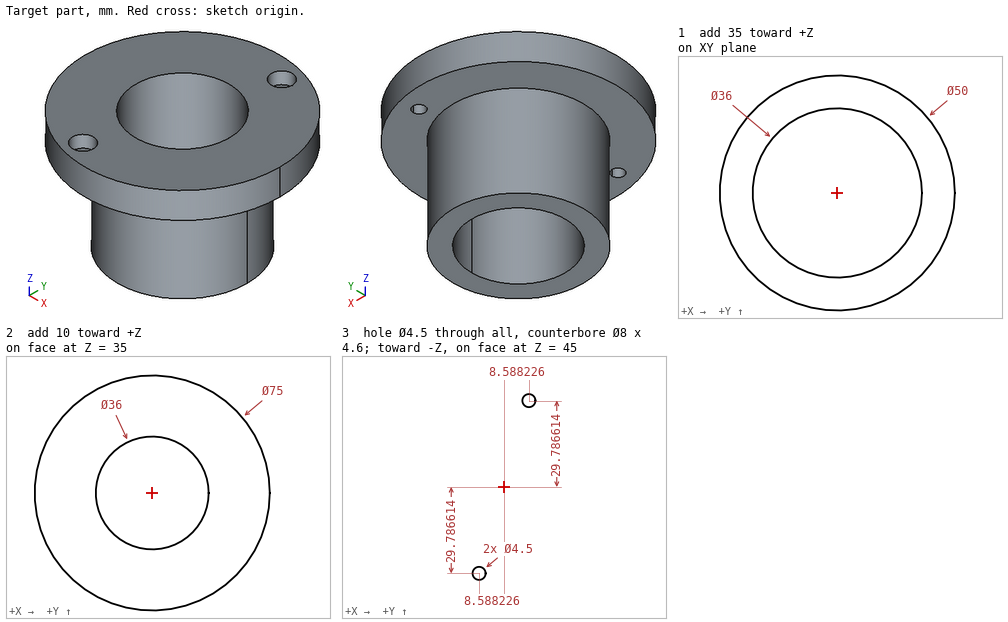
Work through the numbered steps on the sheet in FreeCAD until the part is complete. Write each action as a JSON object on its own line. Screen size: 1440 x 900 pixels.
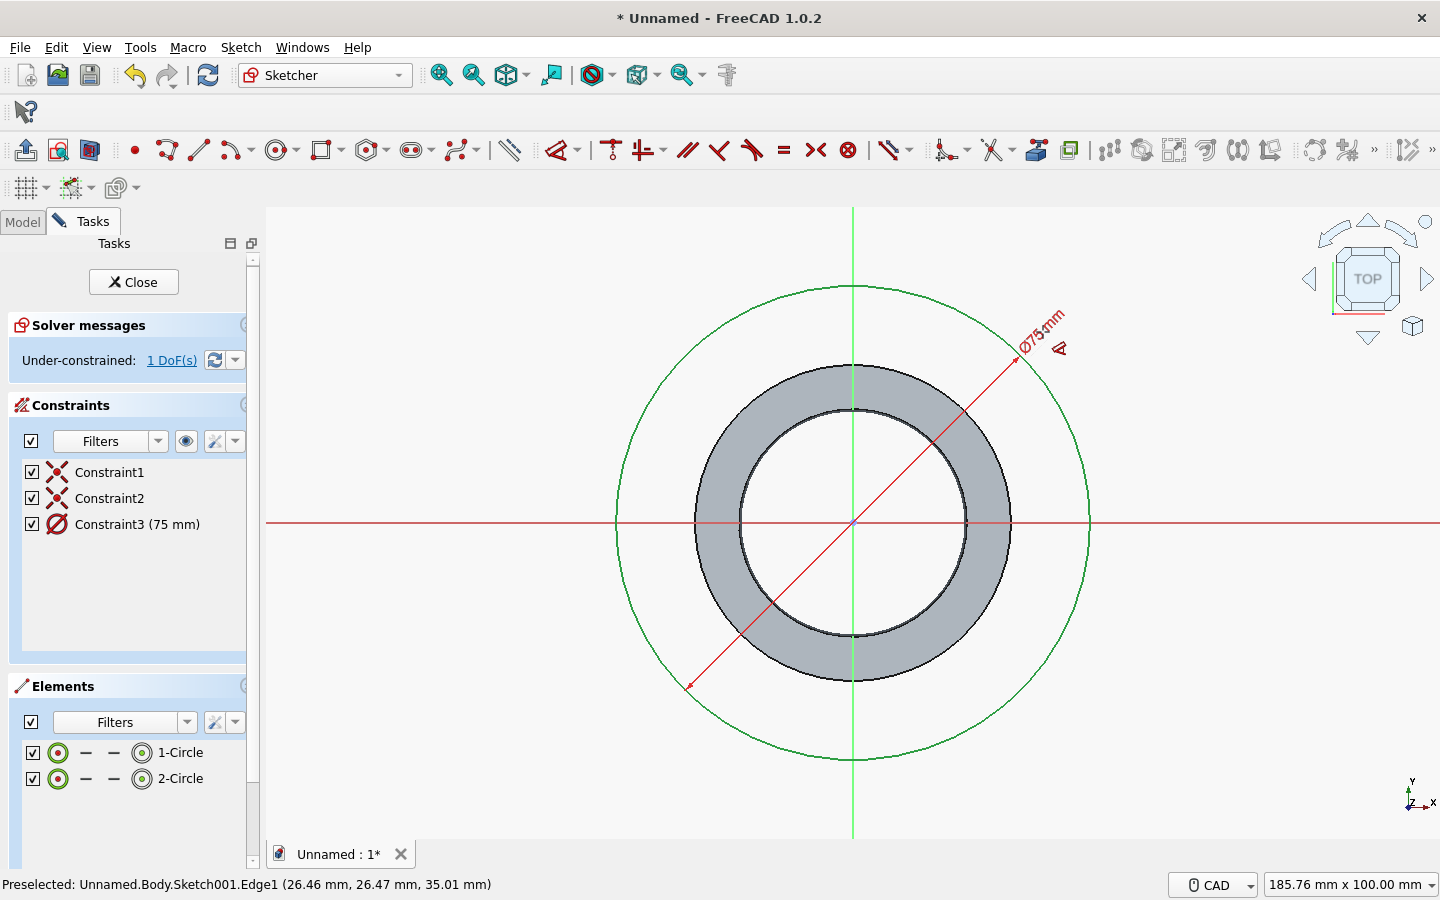
{"action": "left_click", "coordinate": [932, 443]}
{"action": "left_click", "coordinate": [954, 420]}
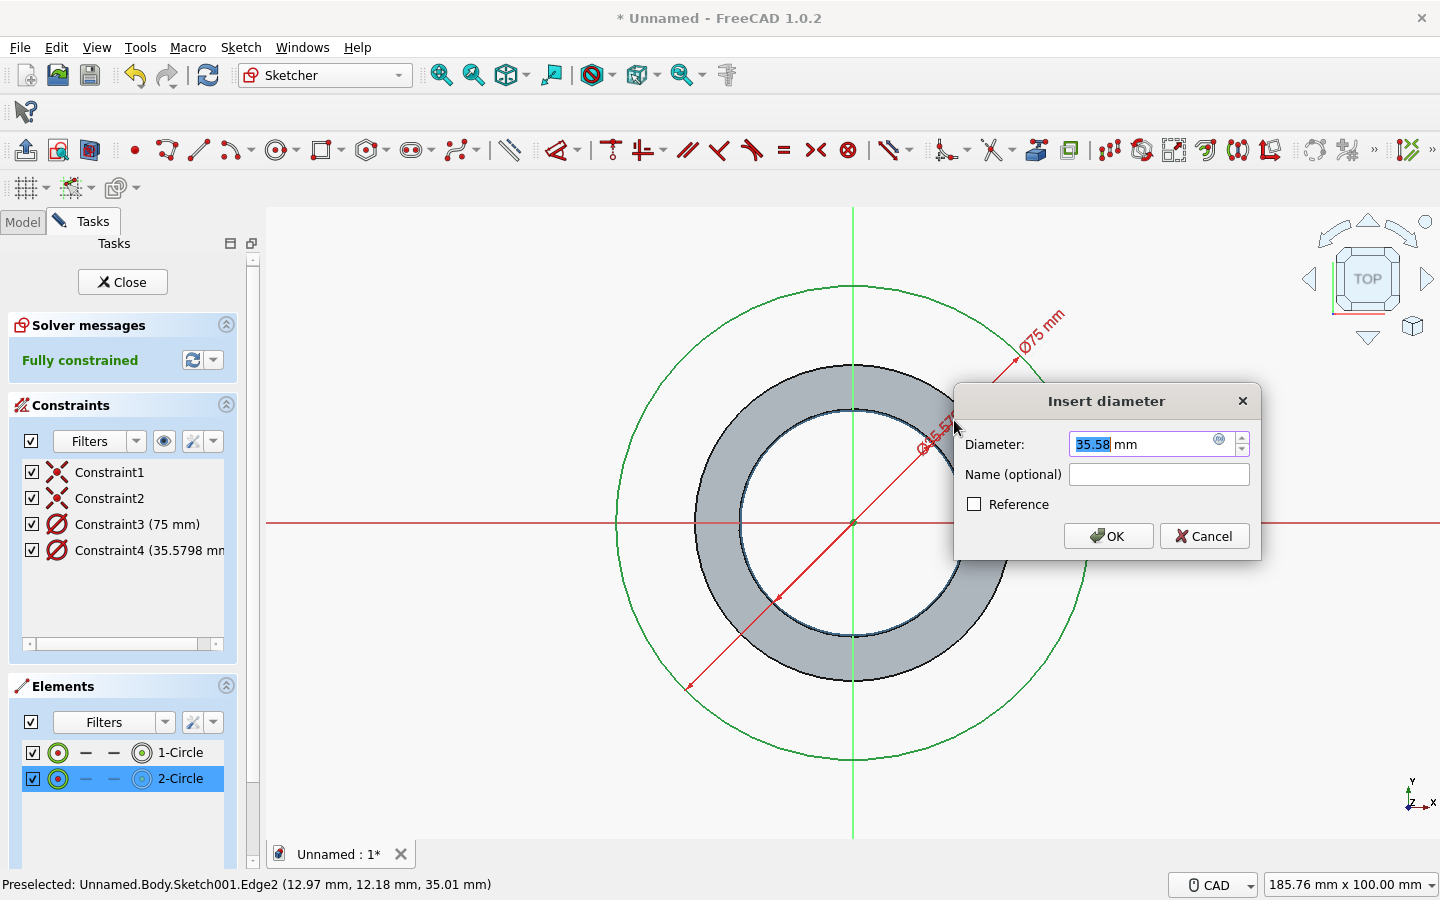
{"action": "type", "text": "36"}
{"action": "key", "text": "Return"}
{"action": "key", "text": "Escape"}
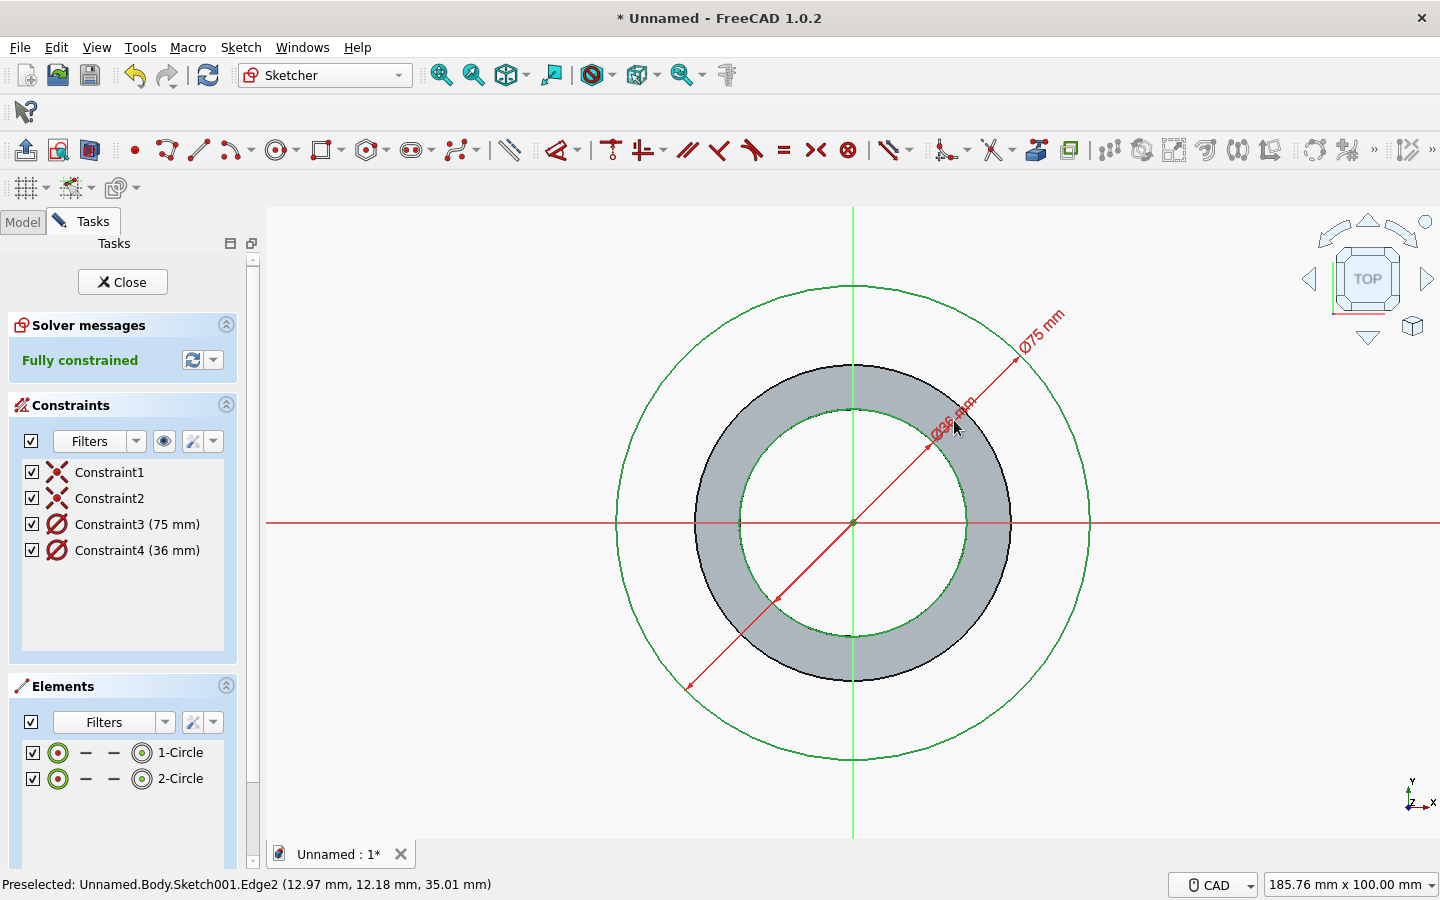
{"action": "left_click", "coordinate": [123, 282]}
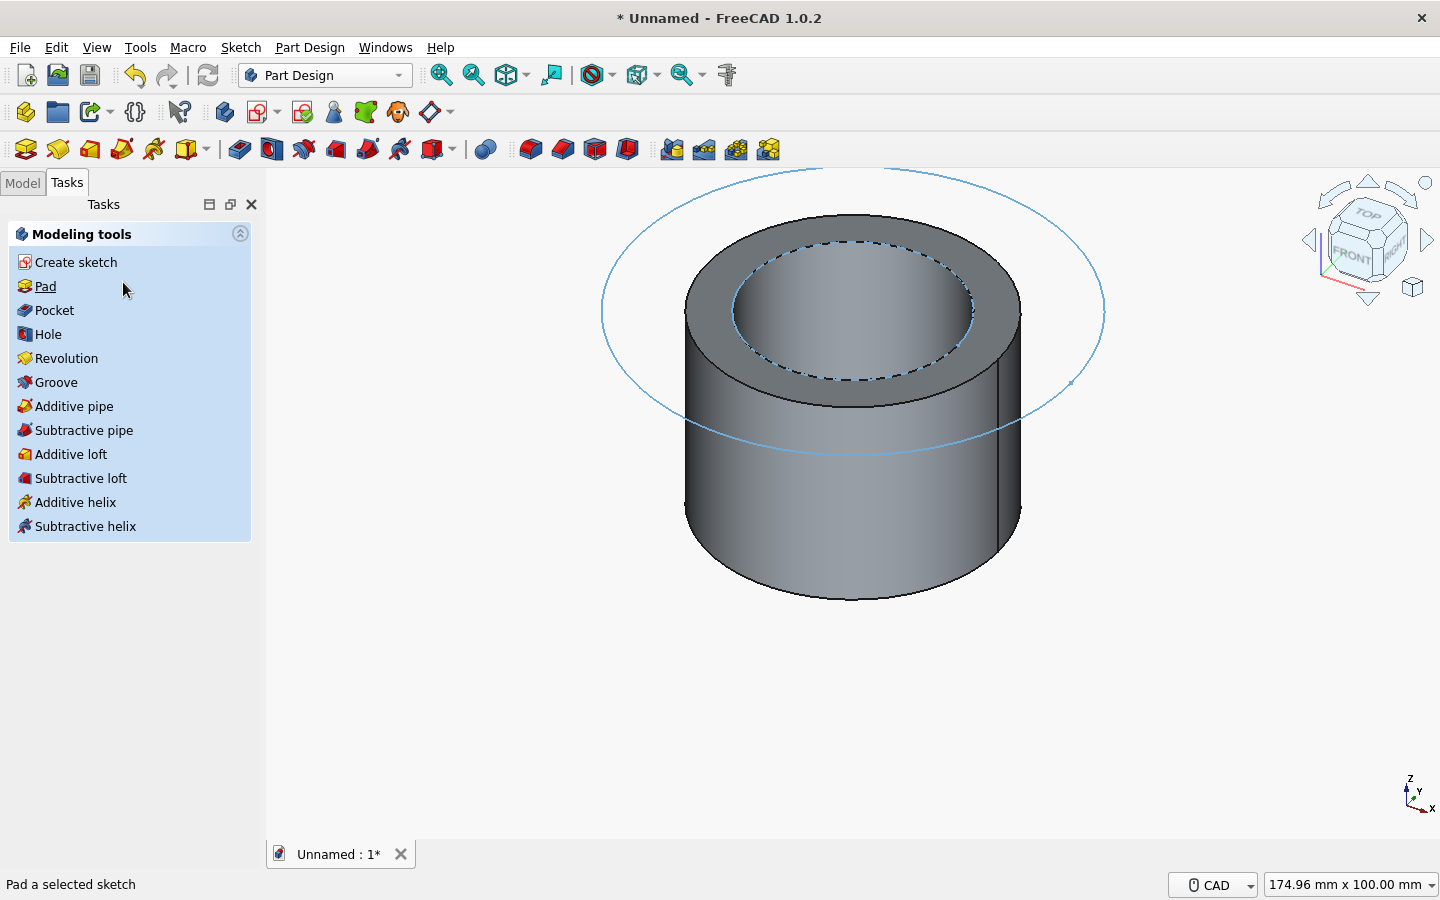
{"action": "left_click", "coordinate": [26, 150]}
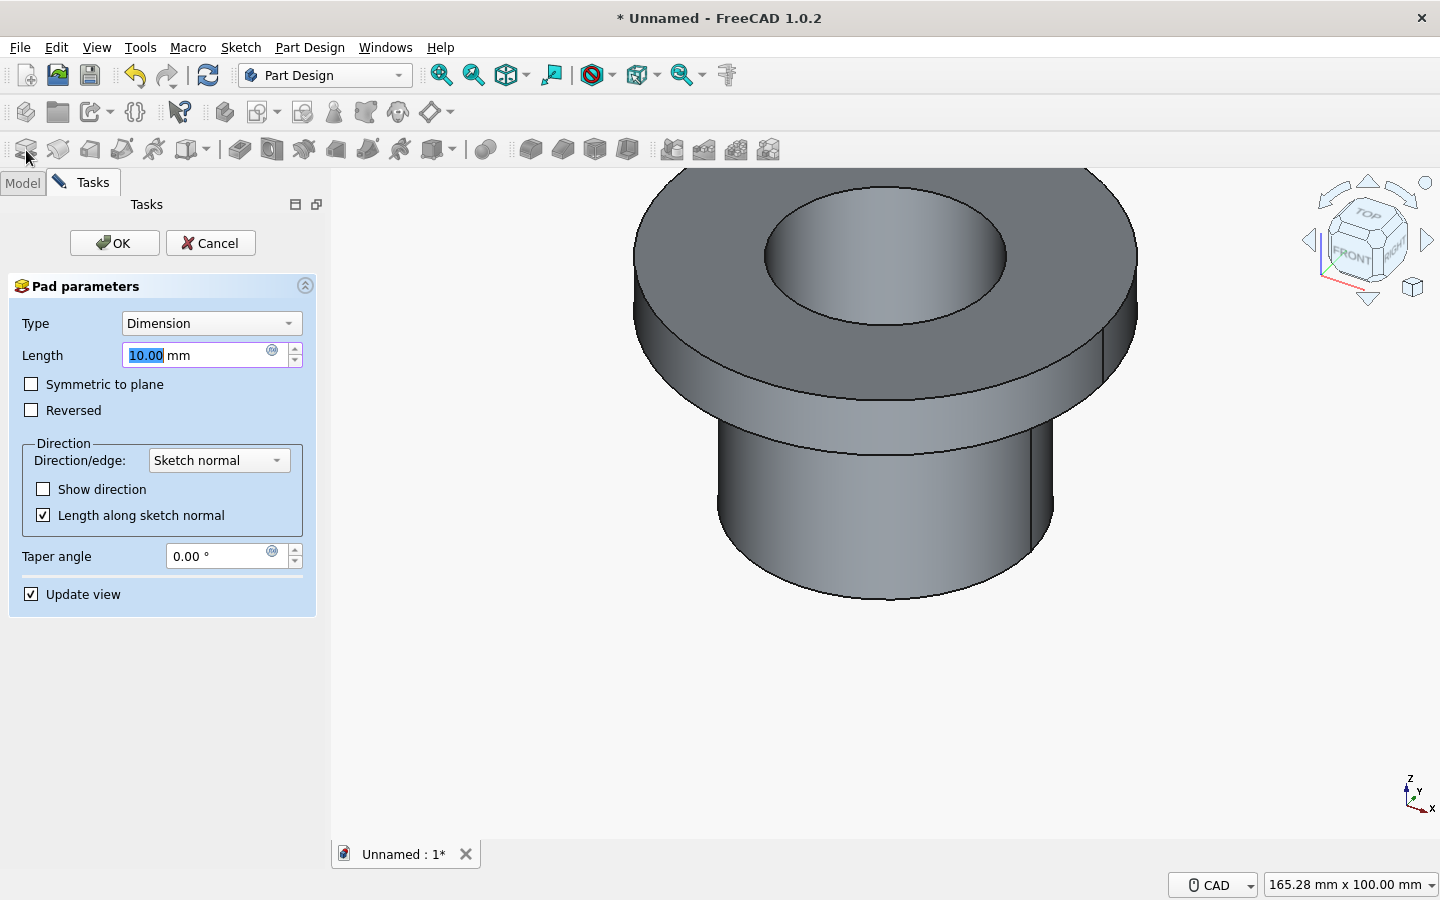
{"action": "type", "text": "10"}
{"action": "key", "text": "Tab"}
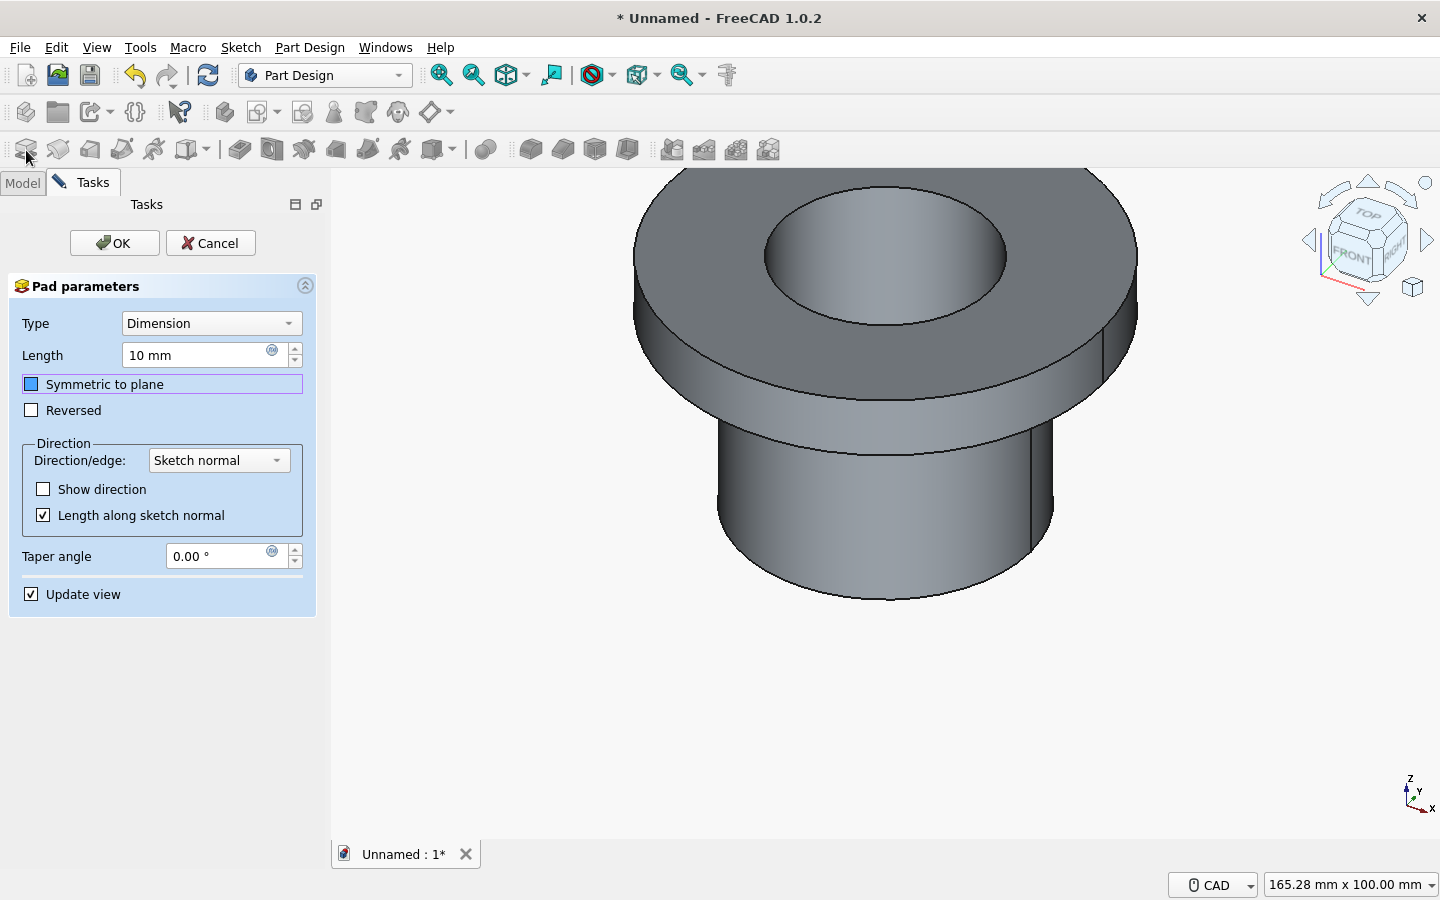
{"action": "left_click", "coordinate": [115, 243]}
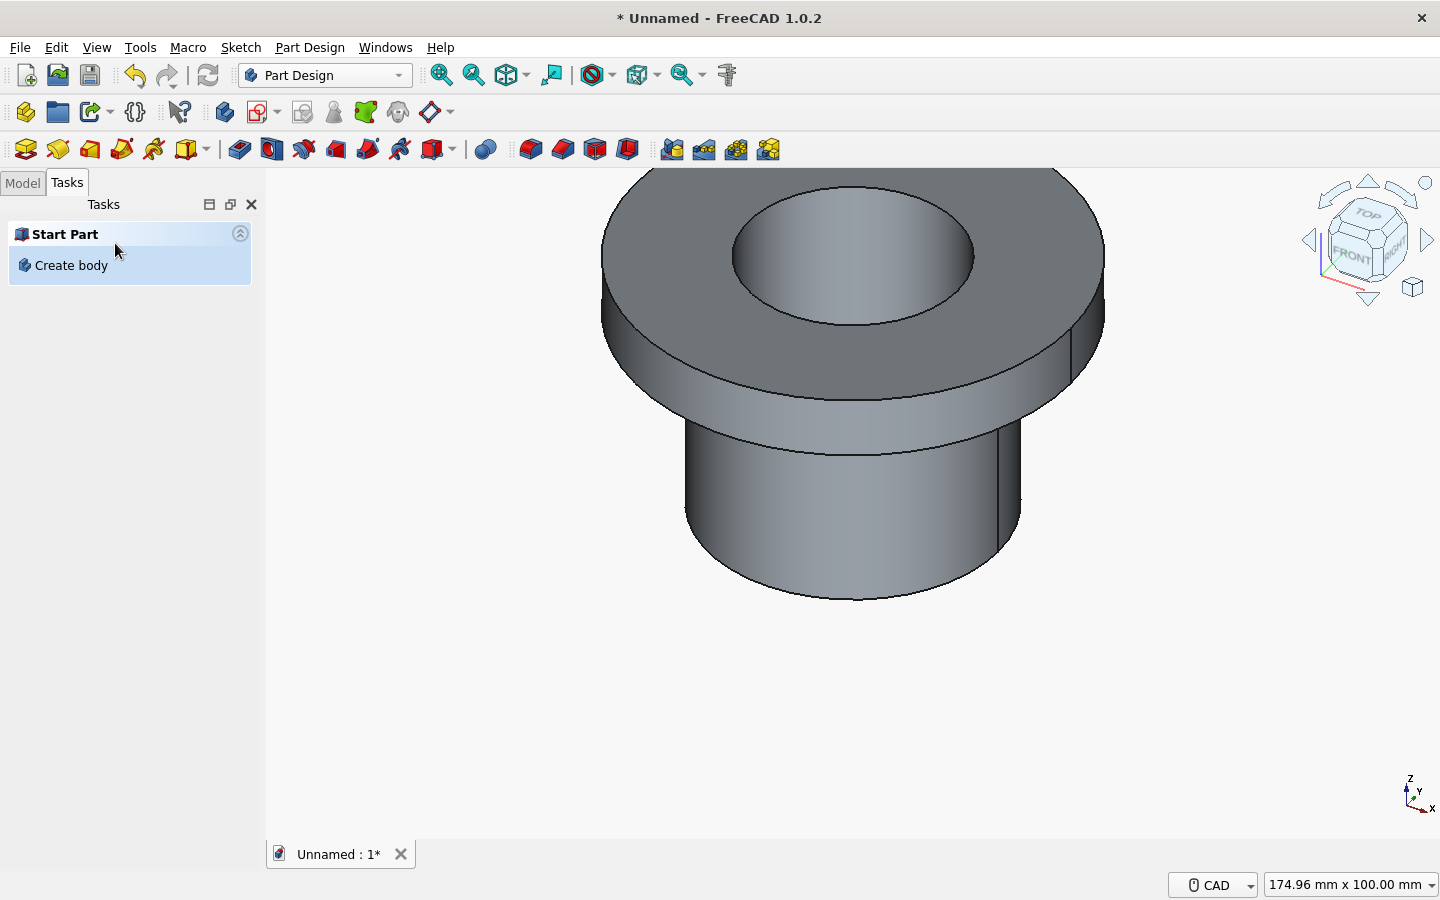
{"action": "key", "text": "v f"}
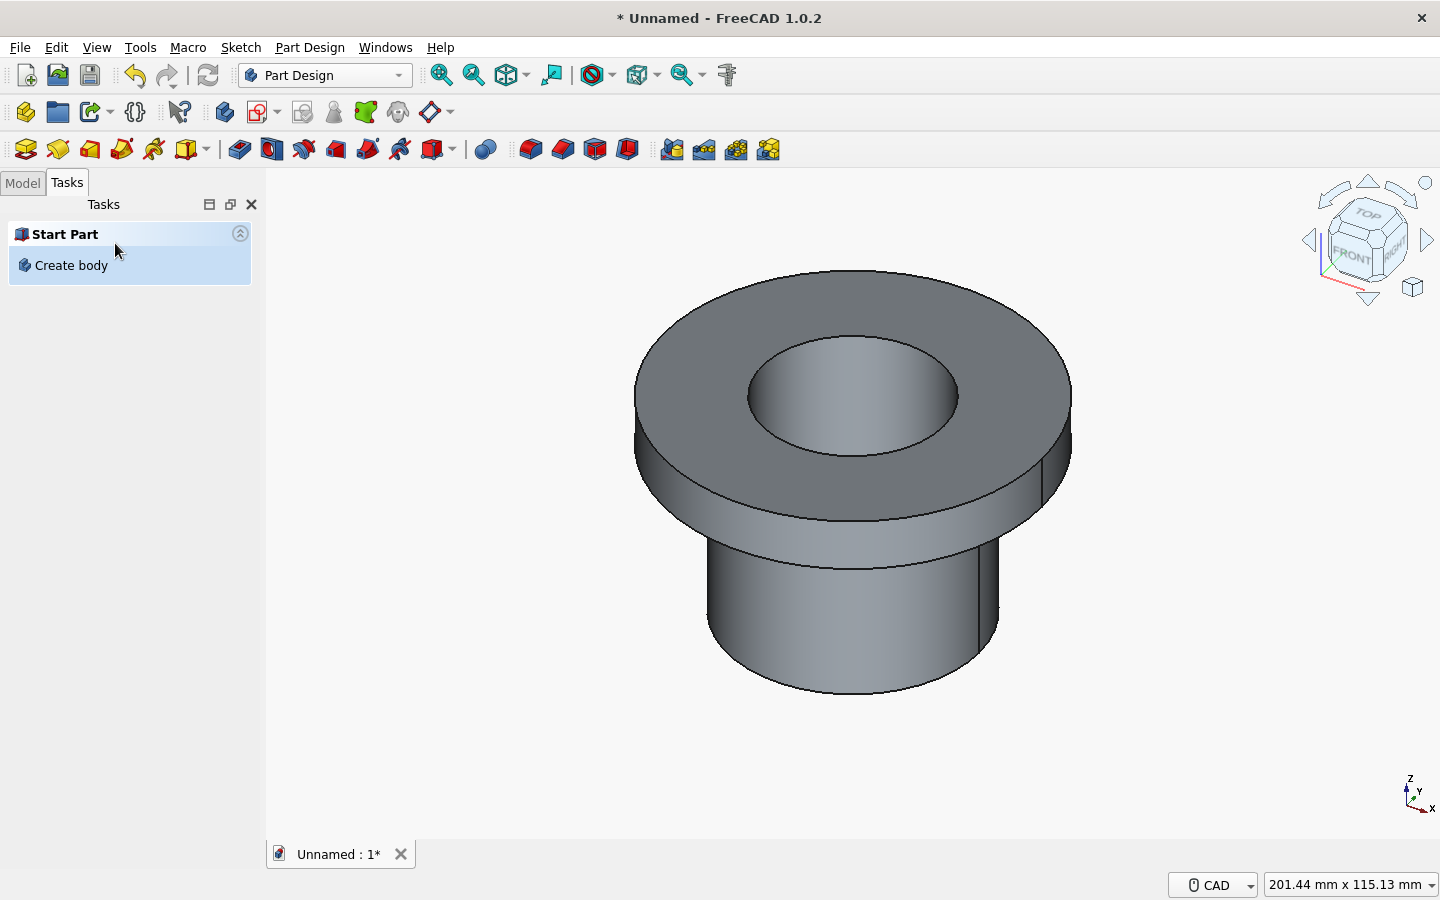
{"action": "left_click", "coordinate": [899, 493]}